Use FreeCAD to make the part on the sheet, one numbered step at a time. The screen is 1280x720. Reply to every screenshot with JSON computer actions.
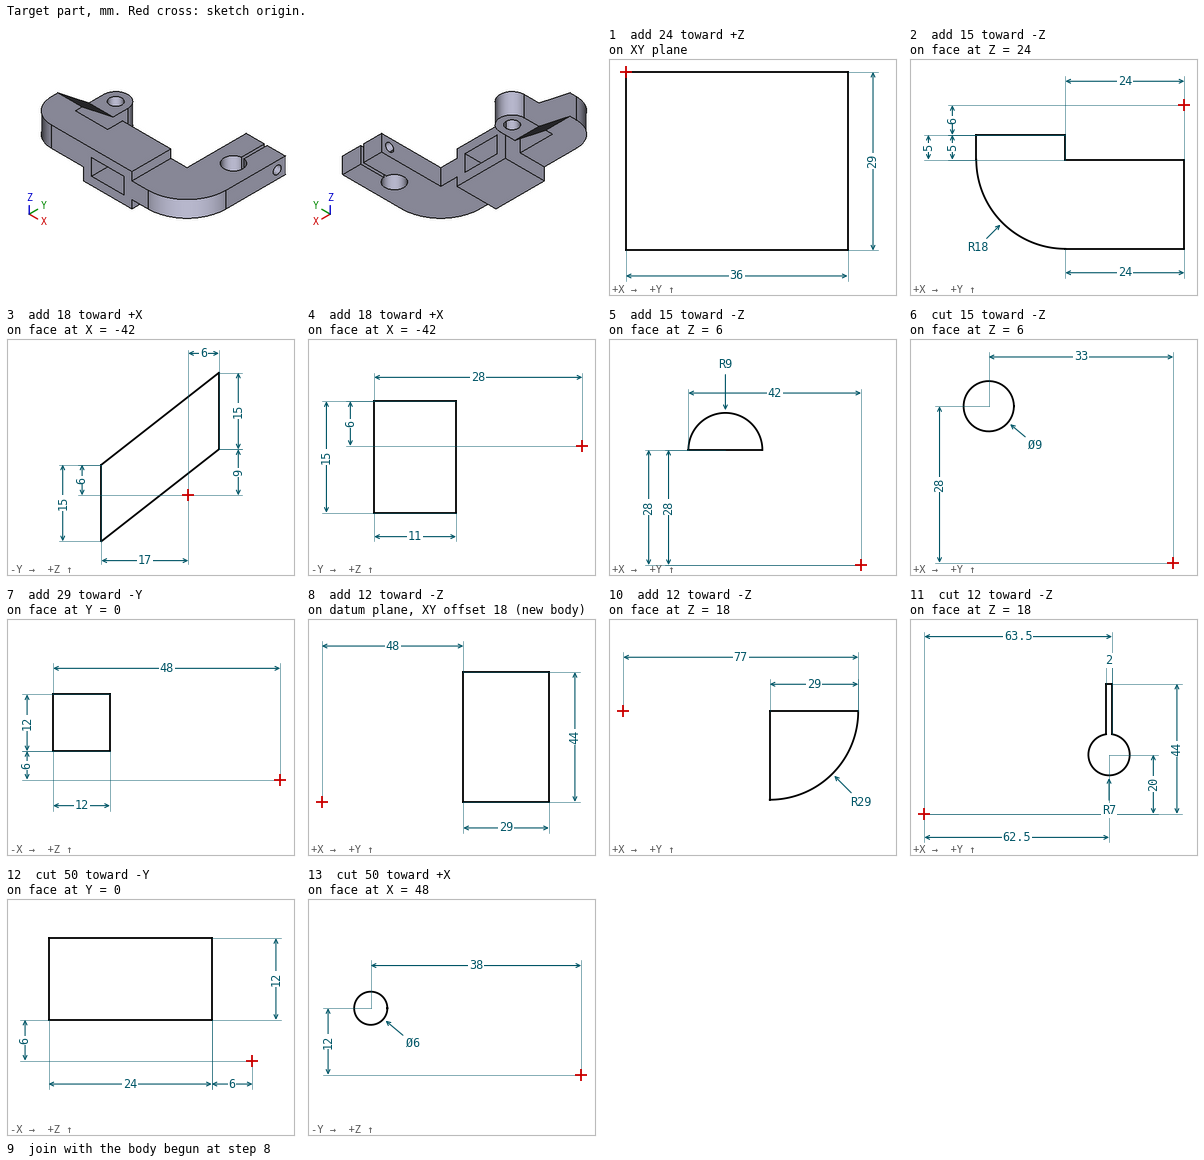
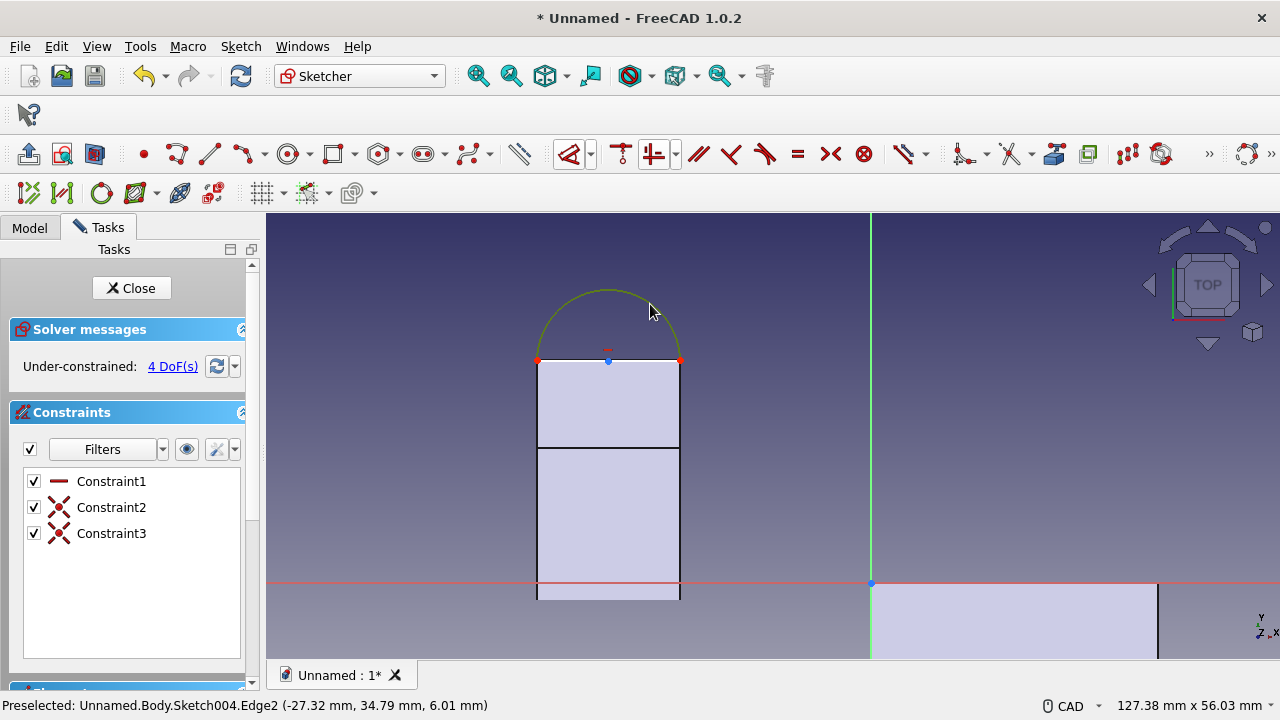
{"action": "left_click", "coordinate": [590, 154]}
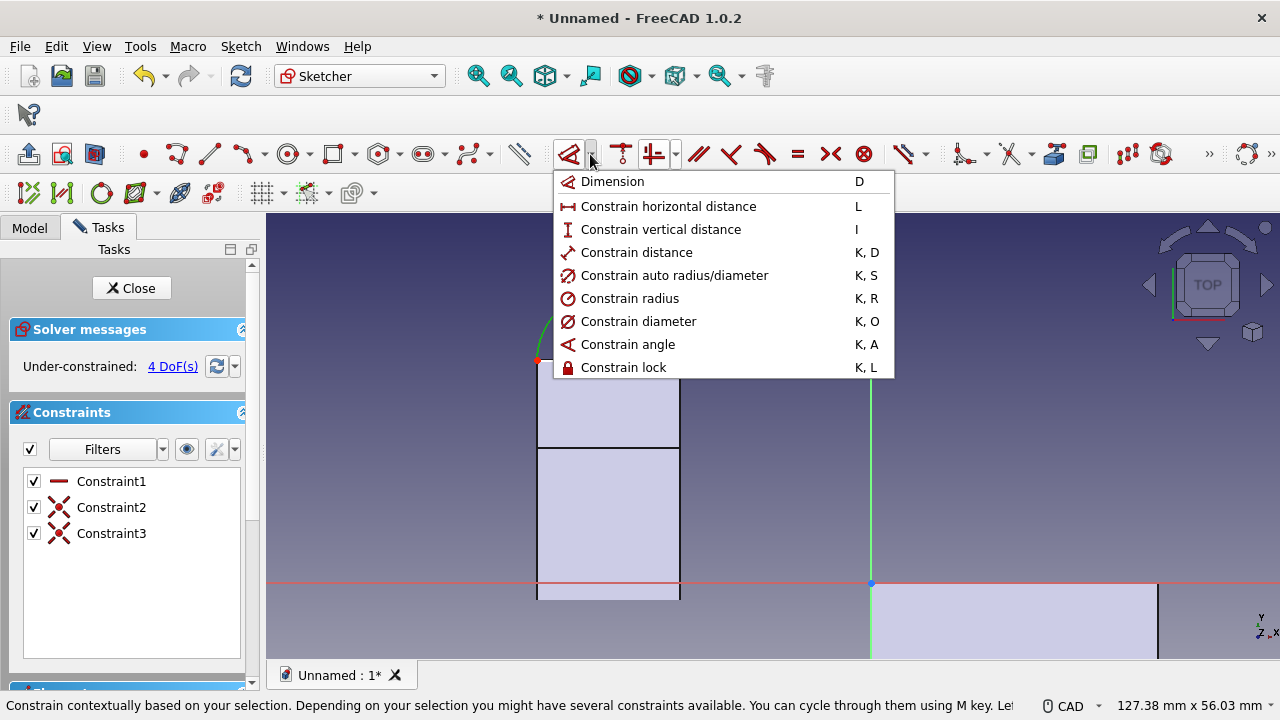
{"action": "left_click", "coordinate": [724, 298]}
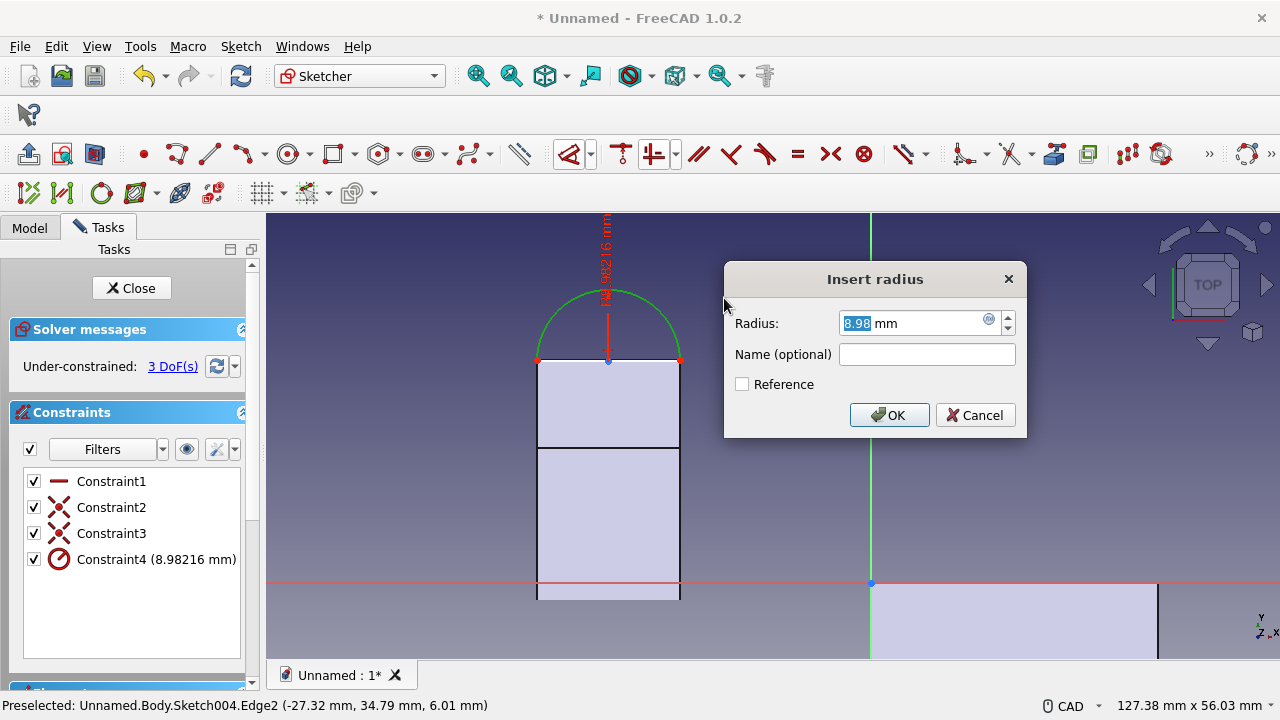
{"action": "type", "text": "9"}
{"action": "key", "text": "Return"}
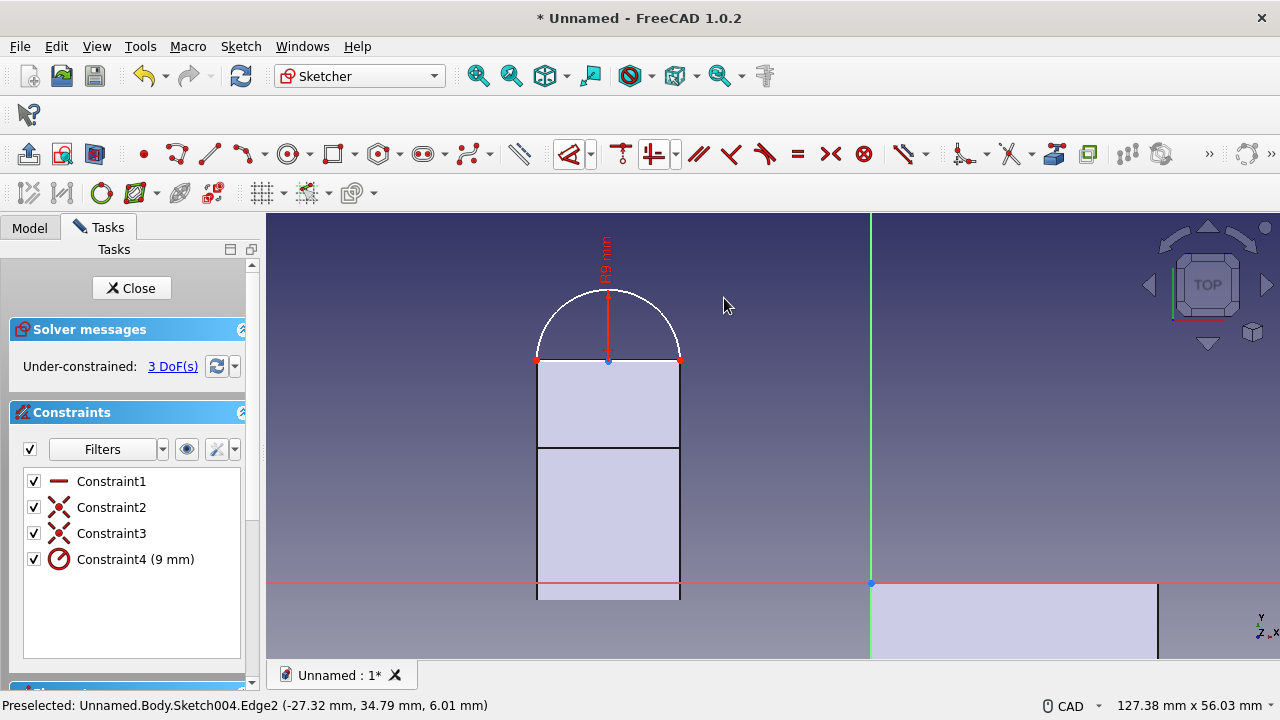
{"action": "left_click", "coordinate": [537, 361]}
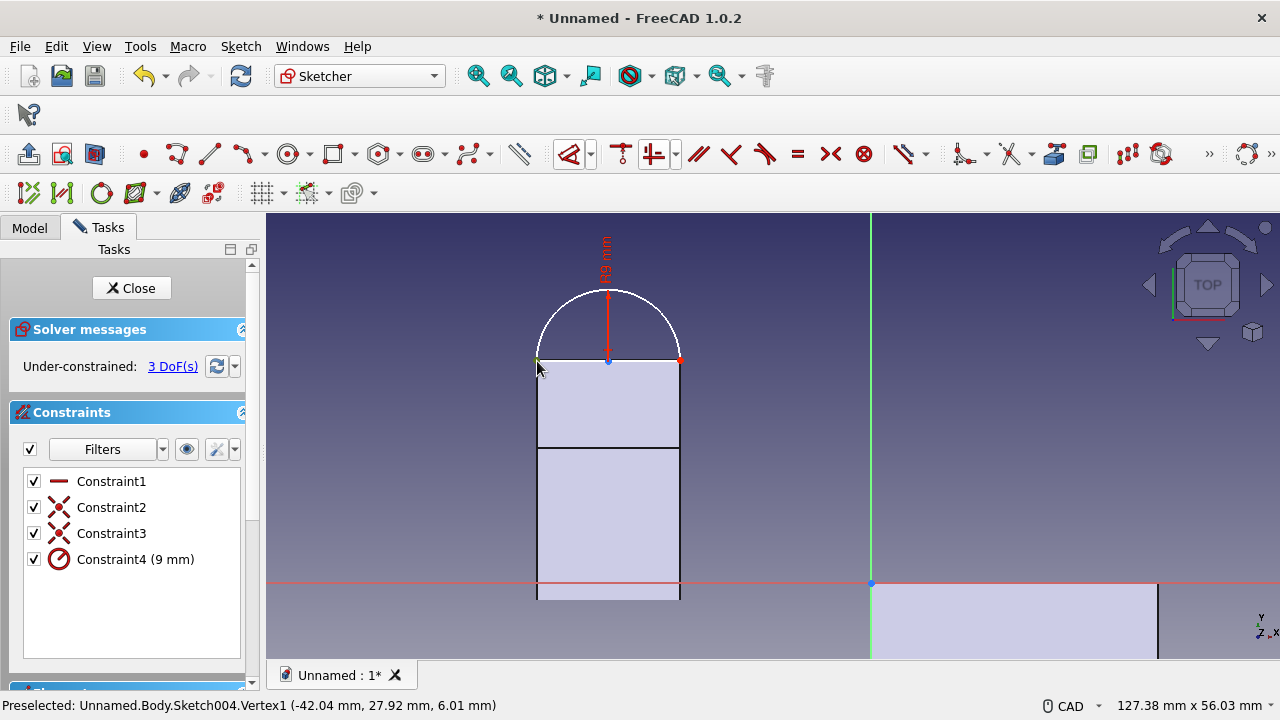
{"action": "left_click", "coordinate": [590, 154]}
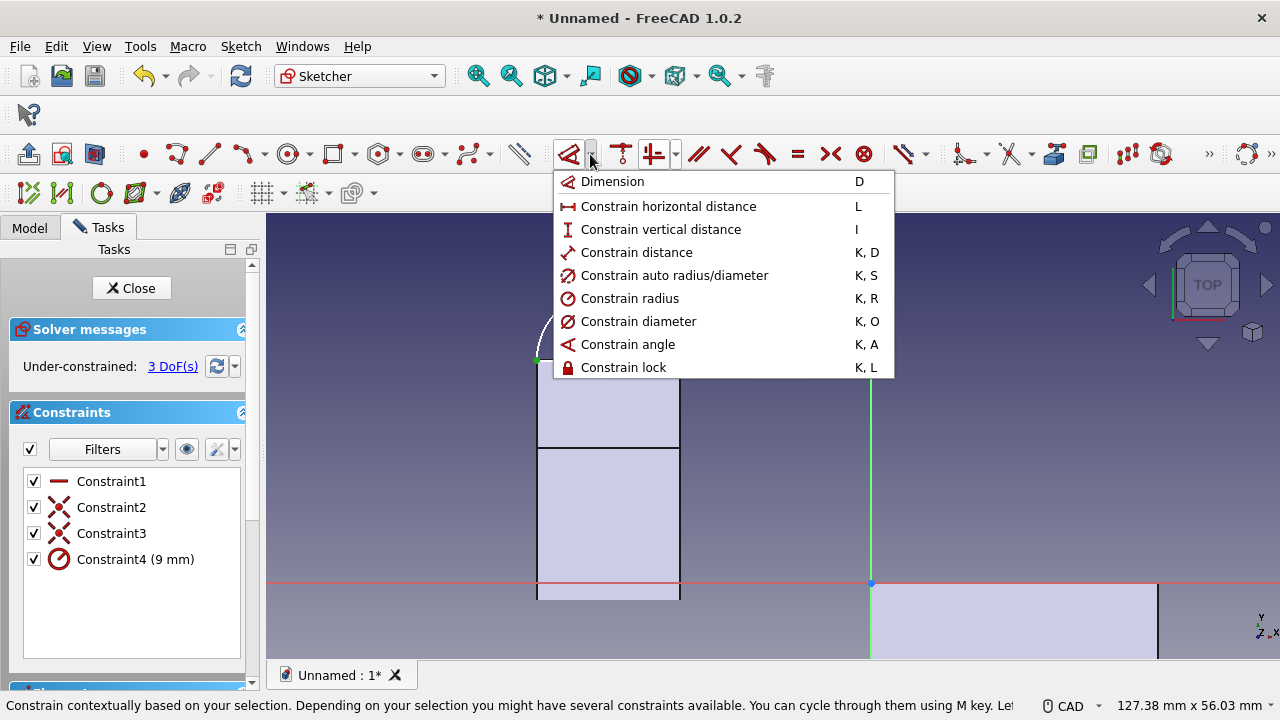
{"action": "left_click", "coordinate": [724, 206]}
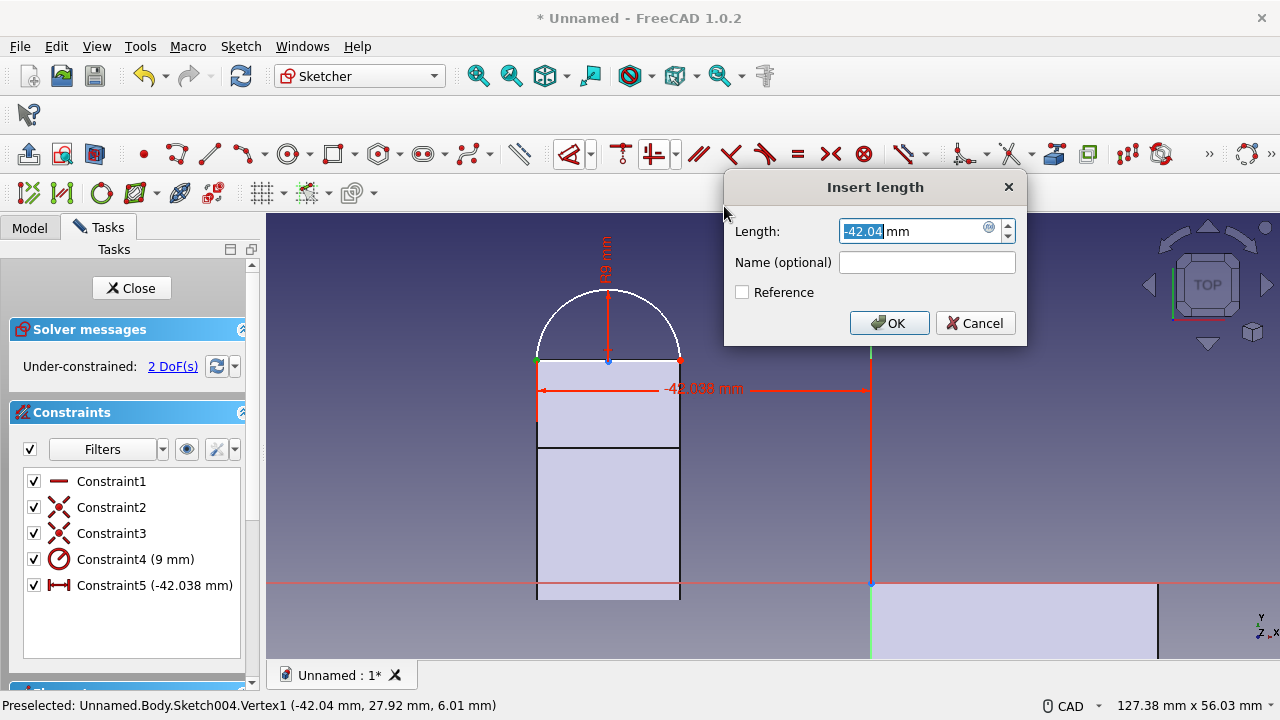
{"action": "type", "text": "-42"}
{"action": "key", "text": "Return"}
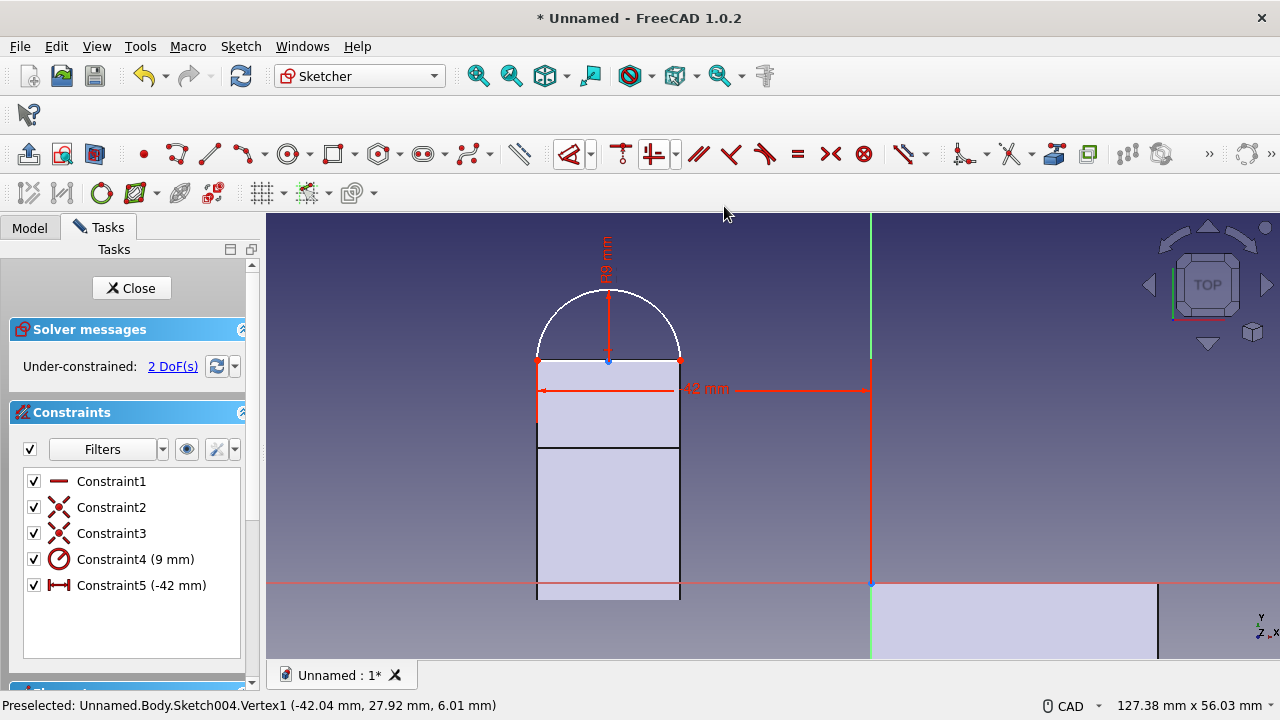
{"action": "left_click", "coordinate": [537, 361]}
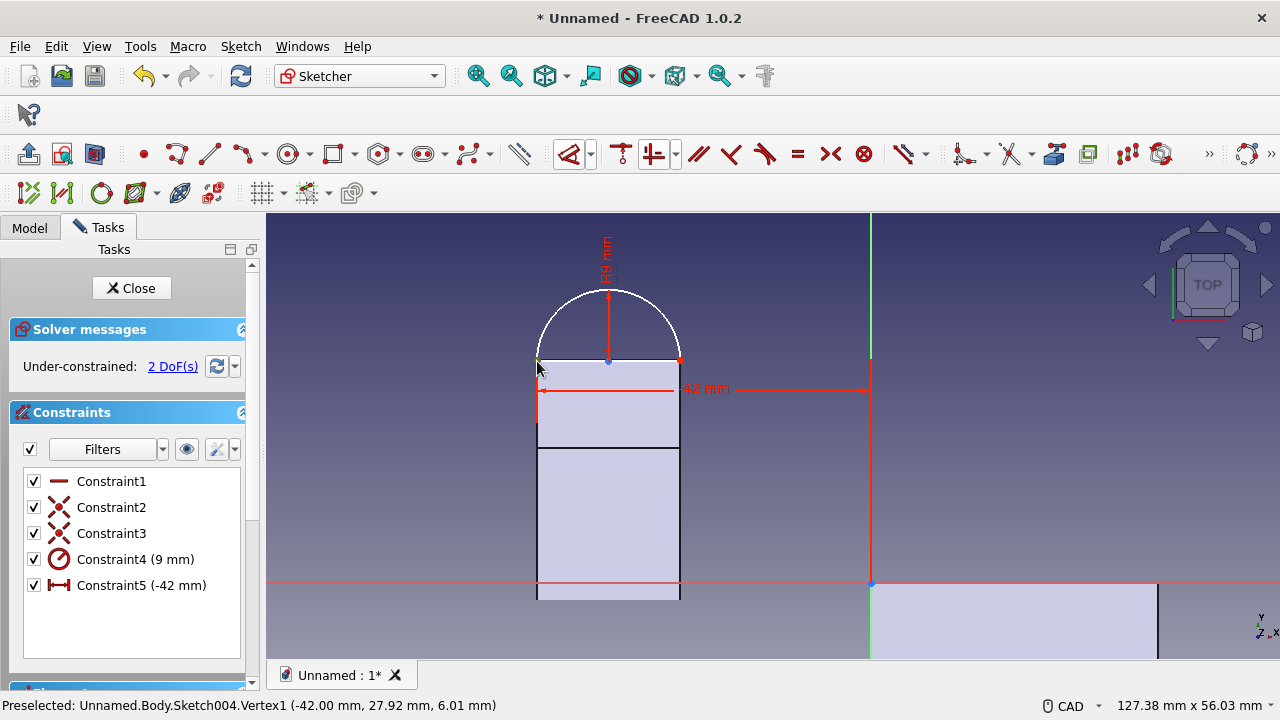
{"action": "left_click", "coordinate": [590, 154]}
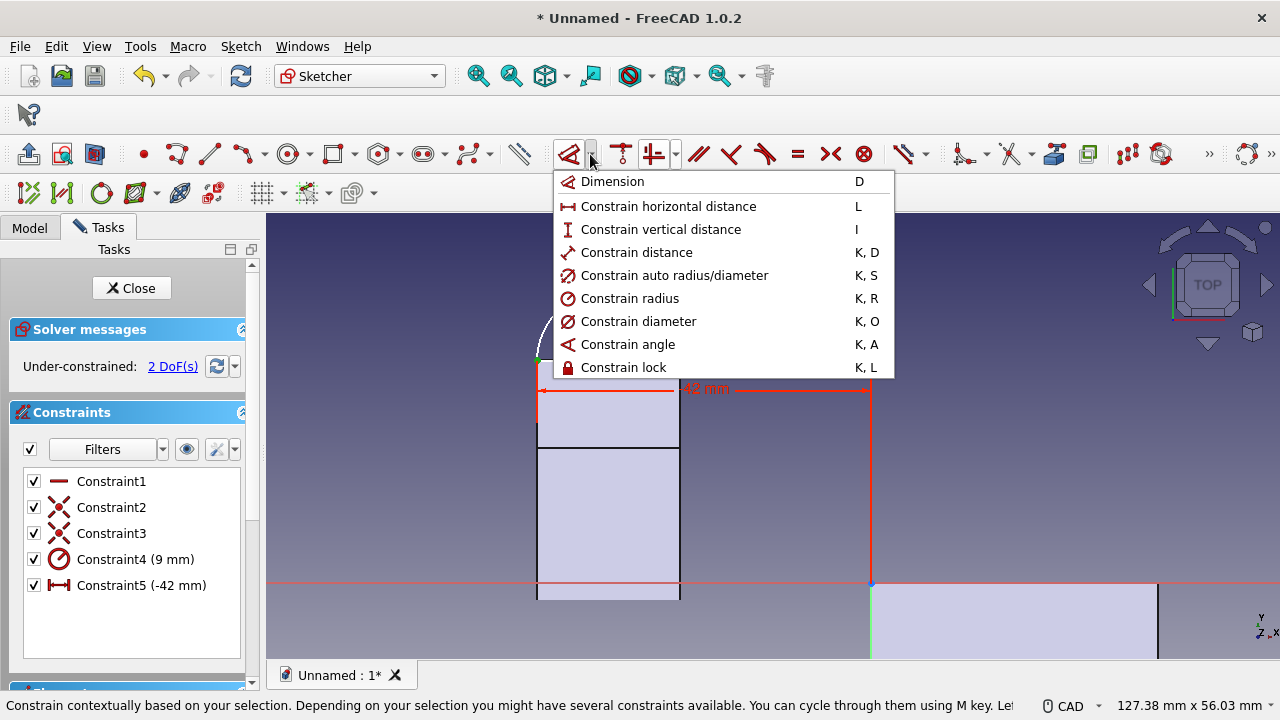
{"action": "left_click", "coordinate": [724, 230]}